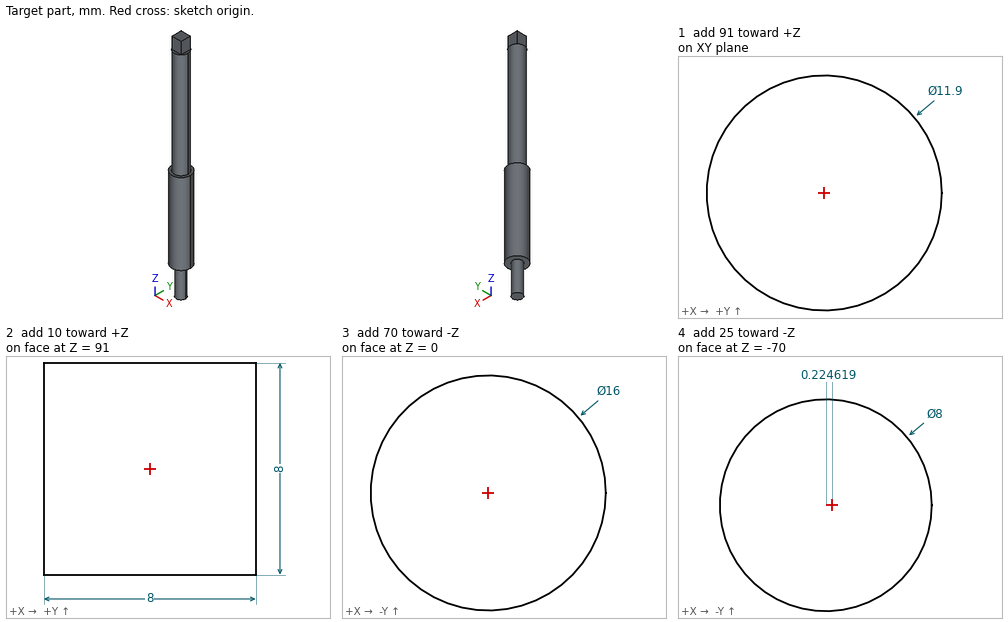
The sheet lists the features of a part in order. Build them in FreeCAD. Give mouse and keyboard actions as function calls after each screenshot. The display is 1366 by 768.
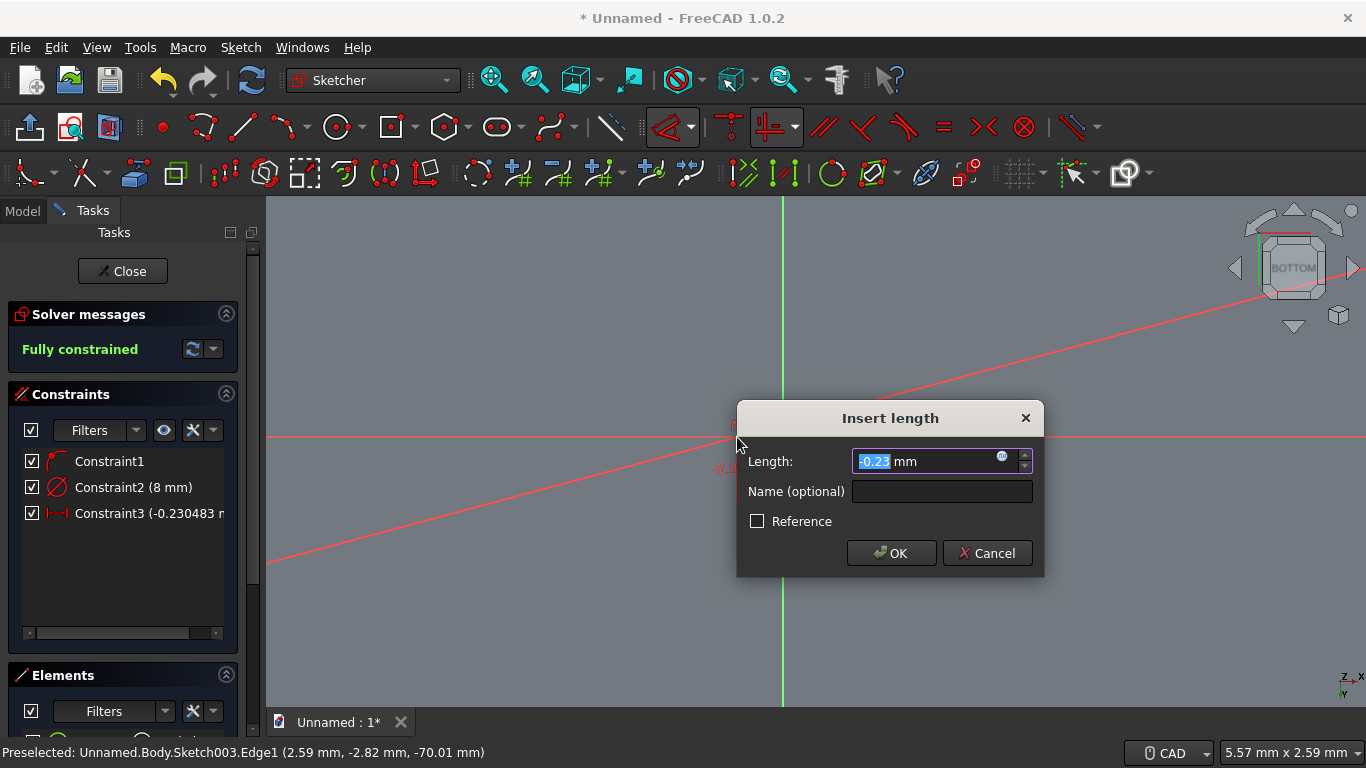
text(-0.224619)
key(Return)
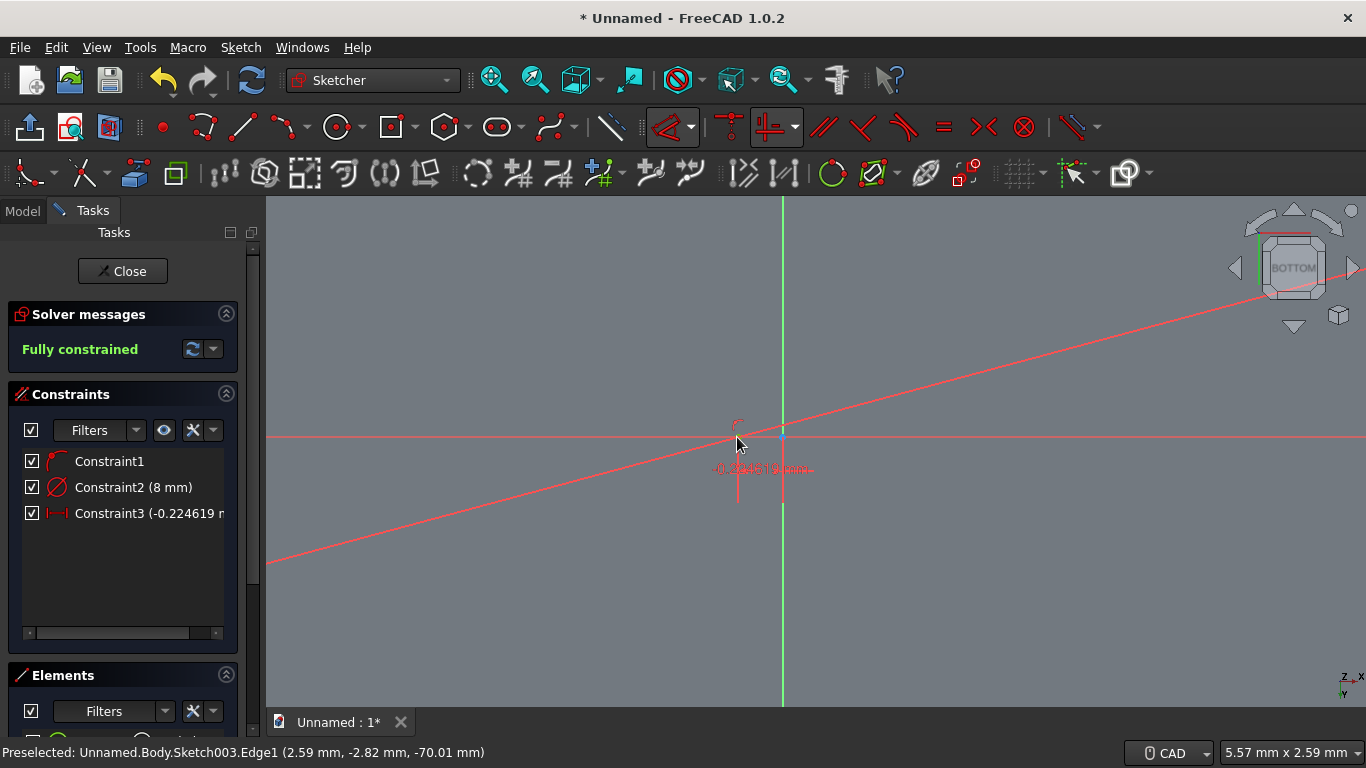
click(123, 271)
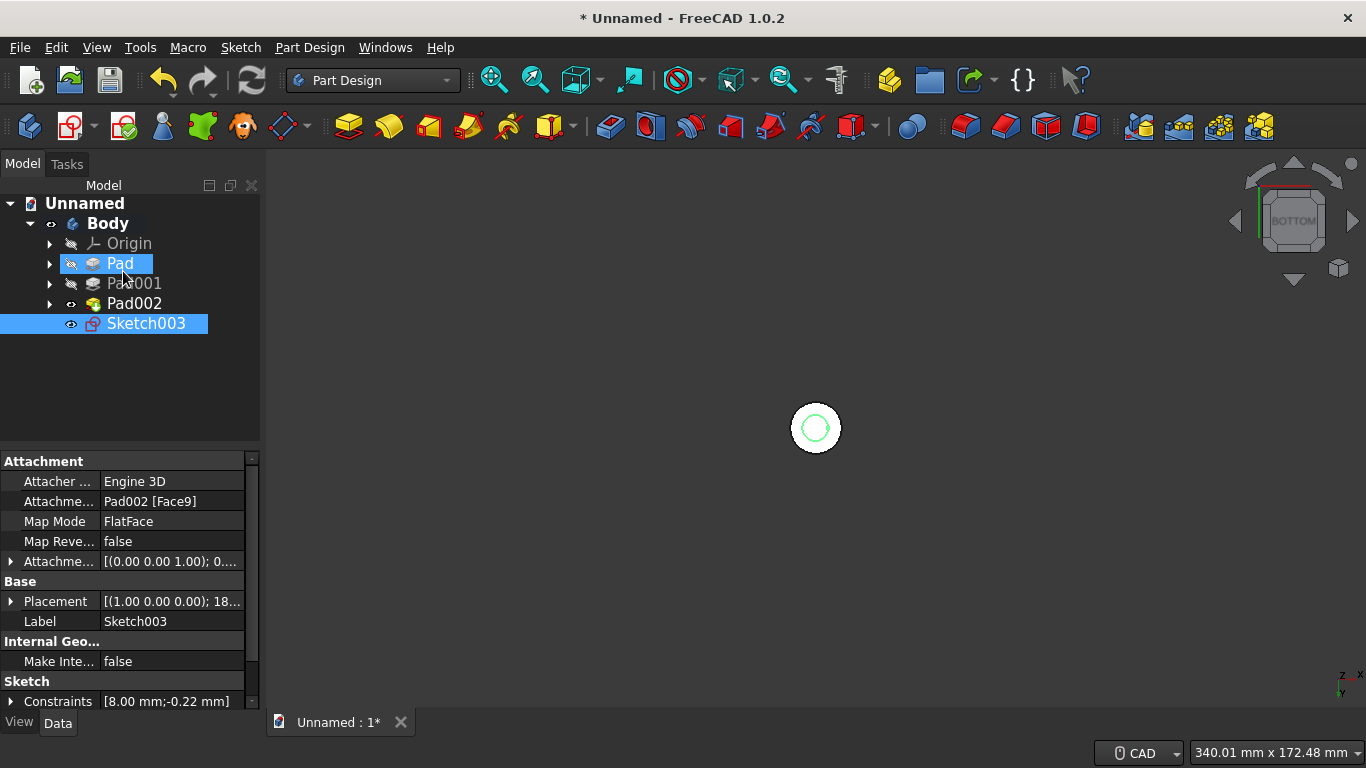
click(350, 126)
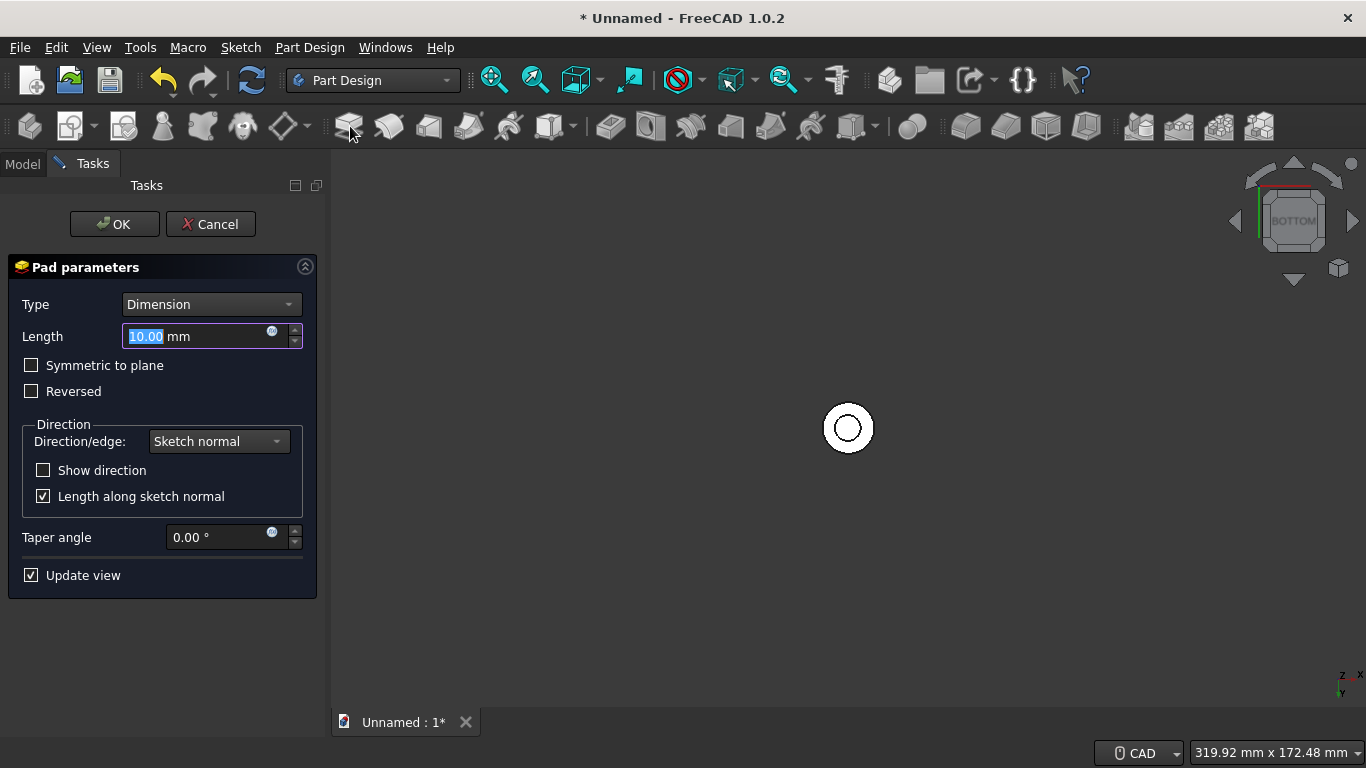
text(25)
key(Tab)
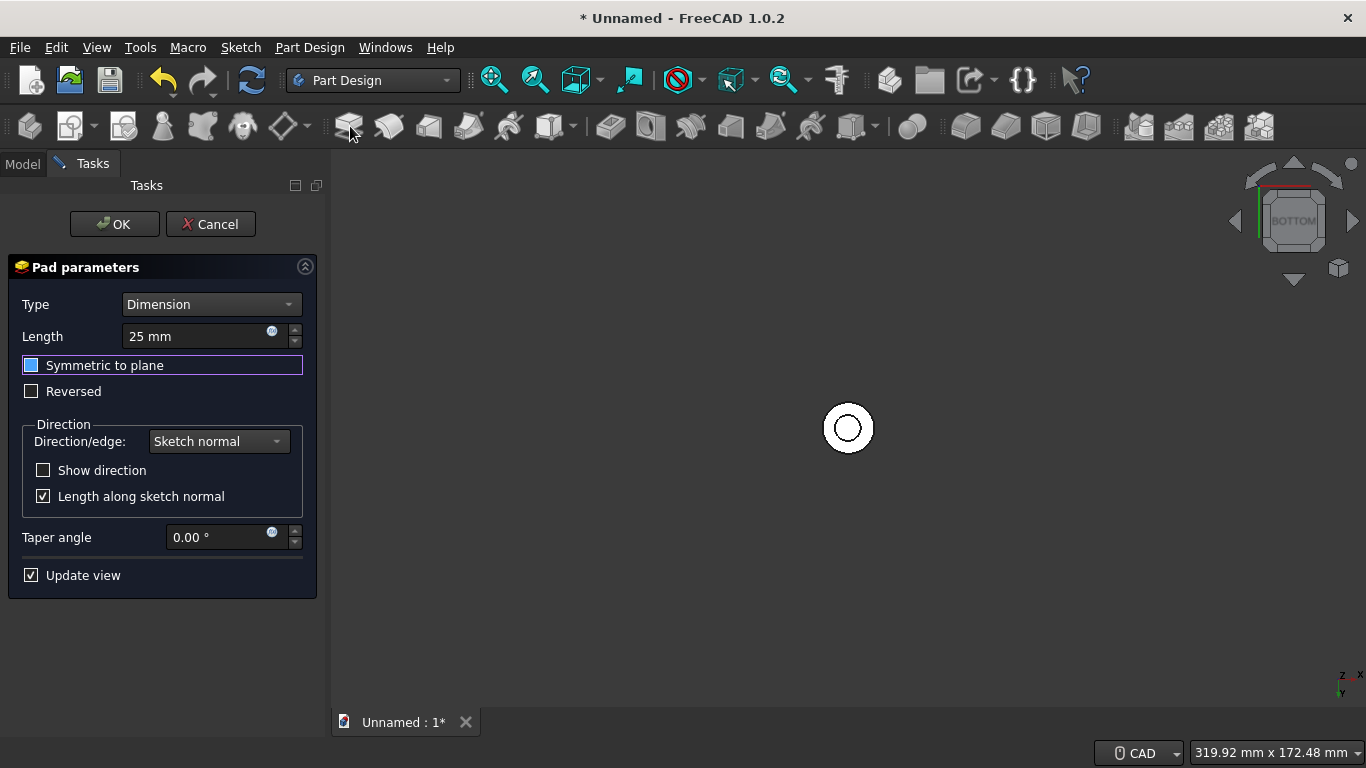
click(115, 224)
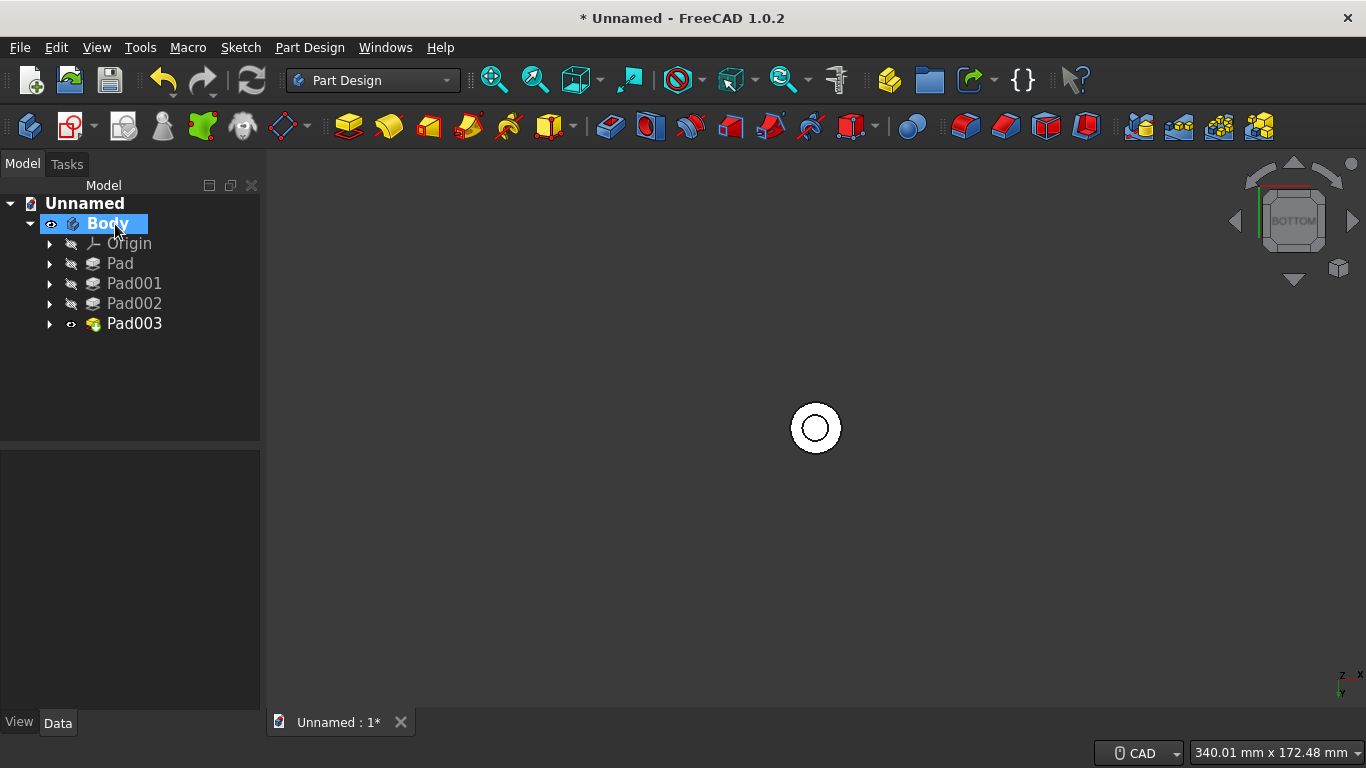
key(0)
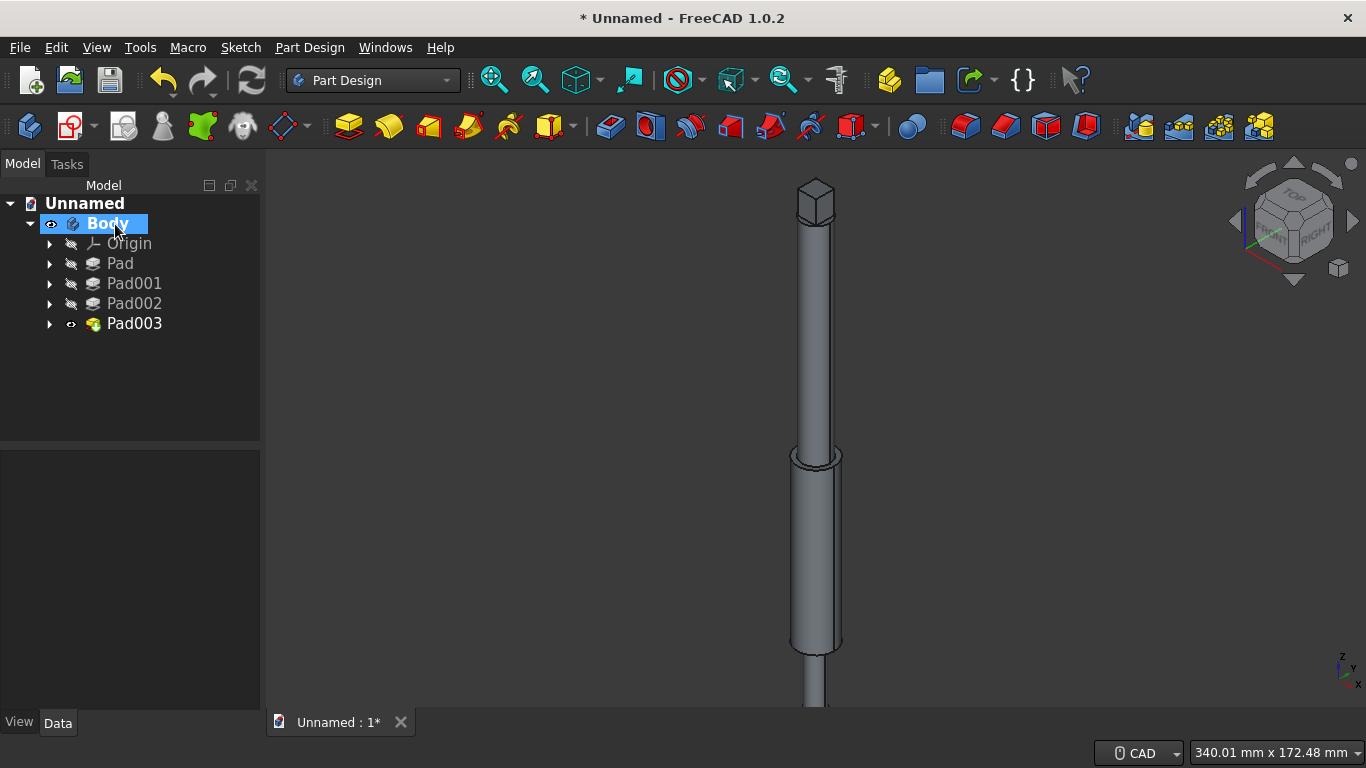
click(496, 80)